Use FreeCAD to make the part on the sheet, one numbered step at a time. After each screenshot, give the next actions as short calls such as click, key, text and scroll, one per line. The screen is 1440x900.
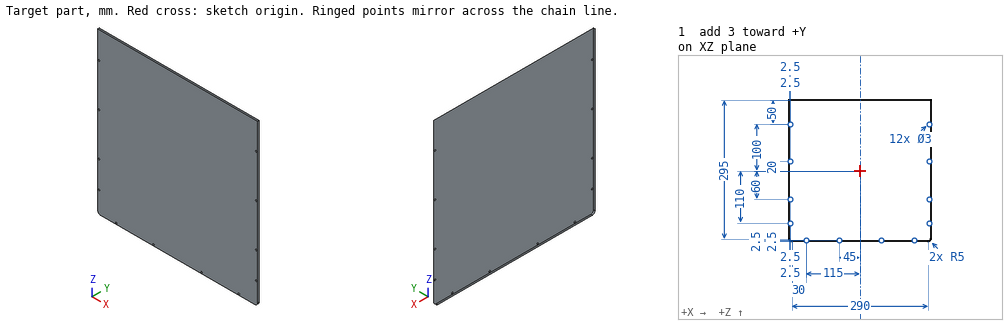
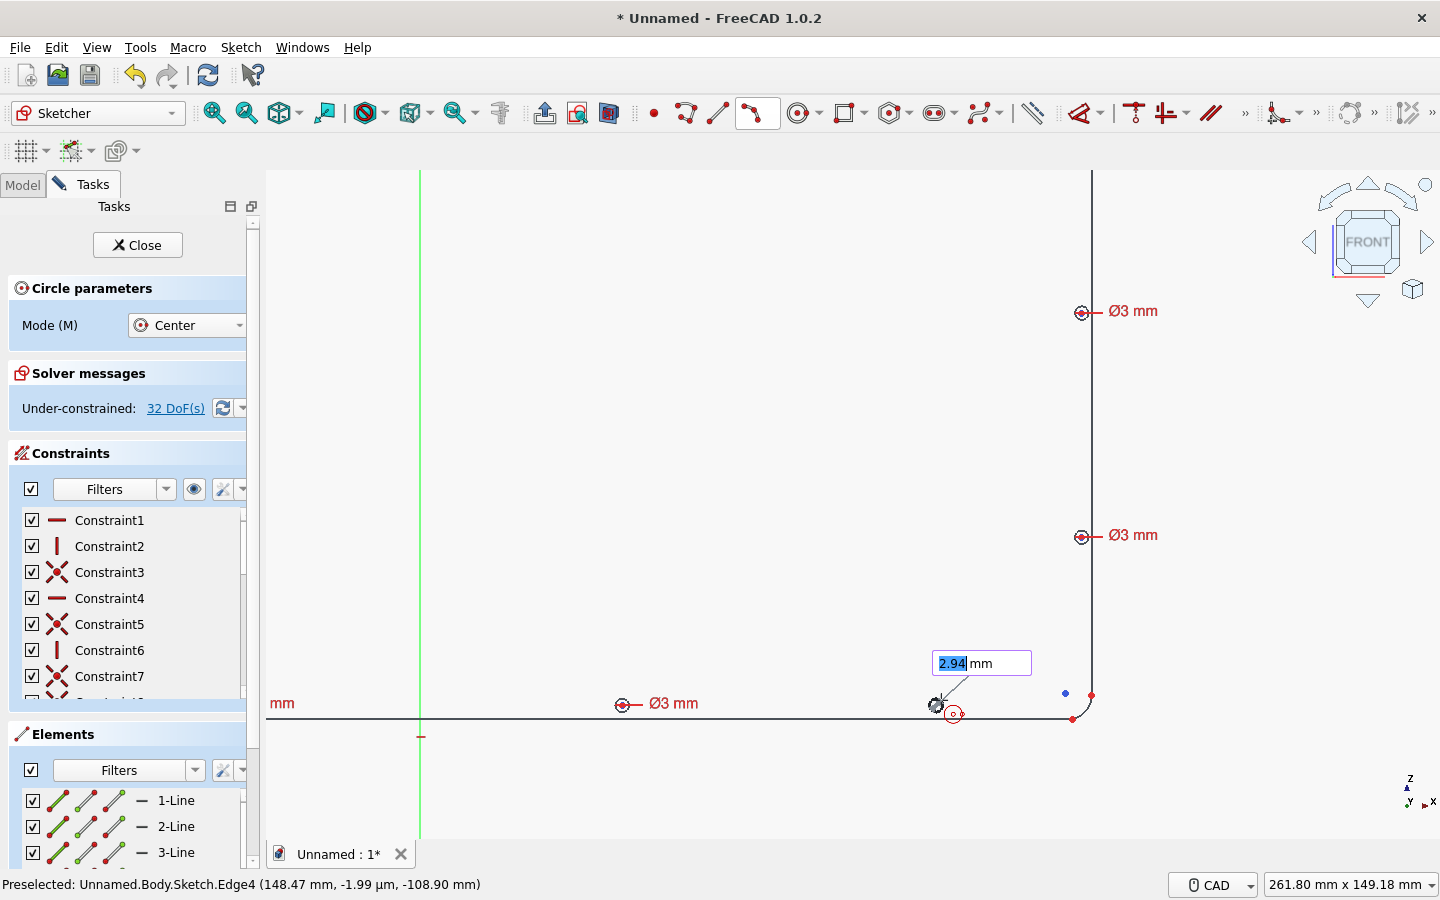
text(3)
key(Return)
key(Escape)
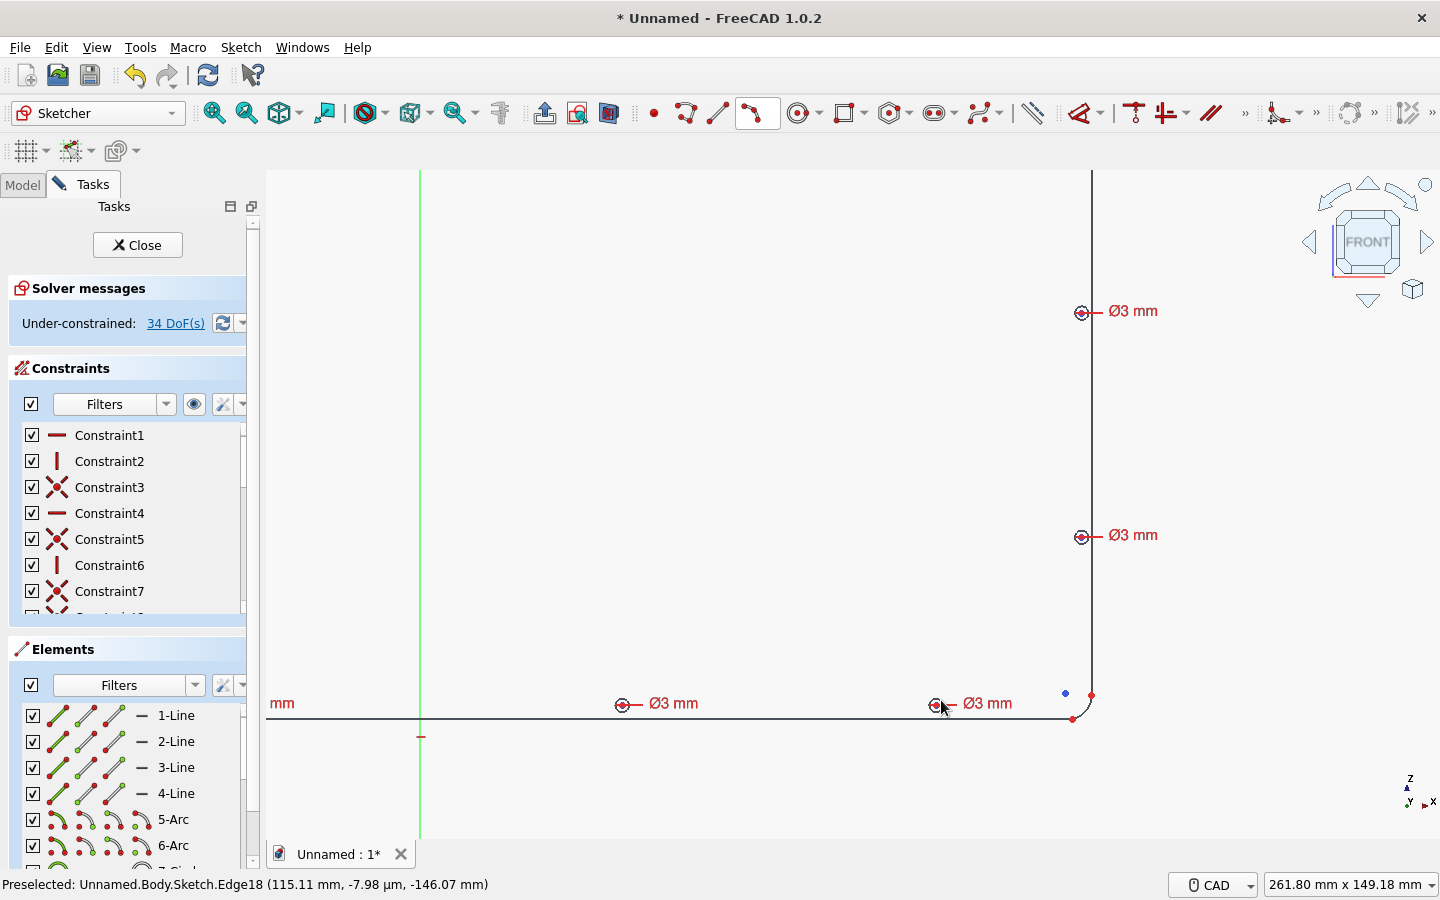
click(682, 719)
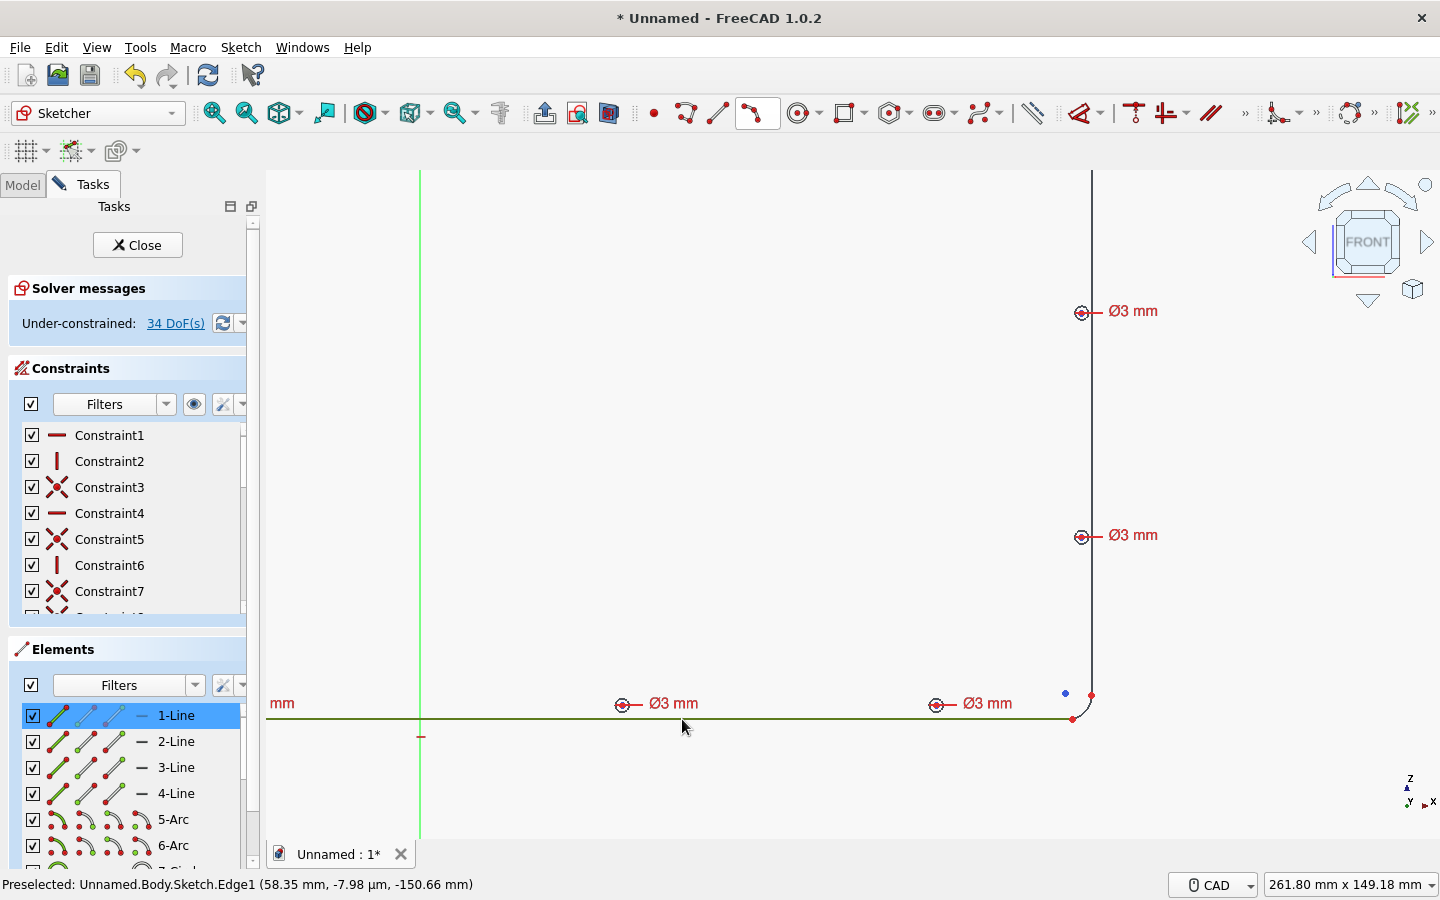
scroll(941, 703, down, 6)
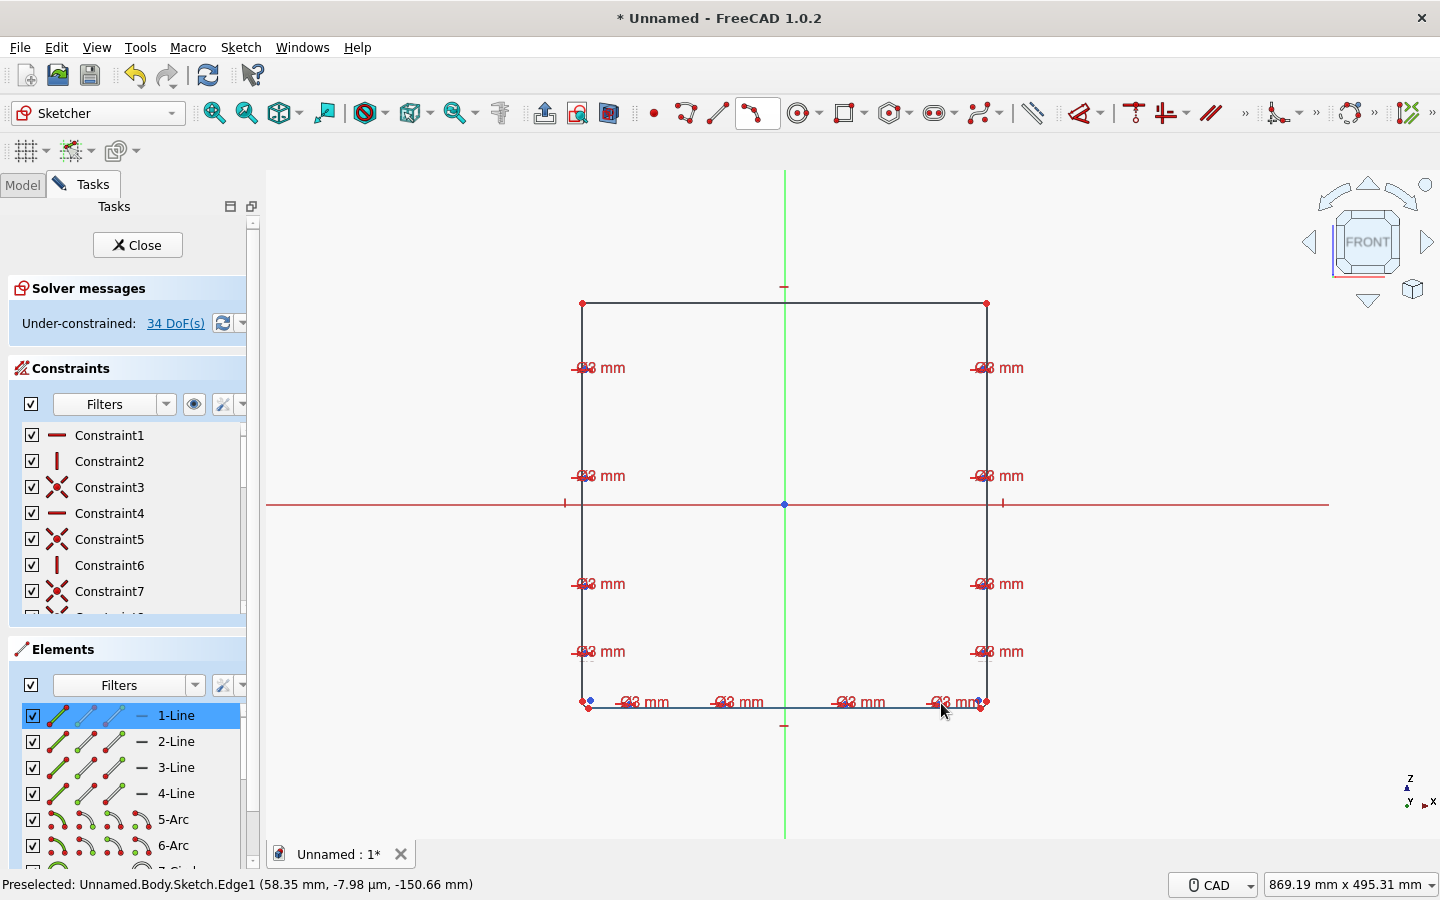
scroll(583, 704, up, 8)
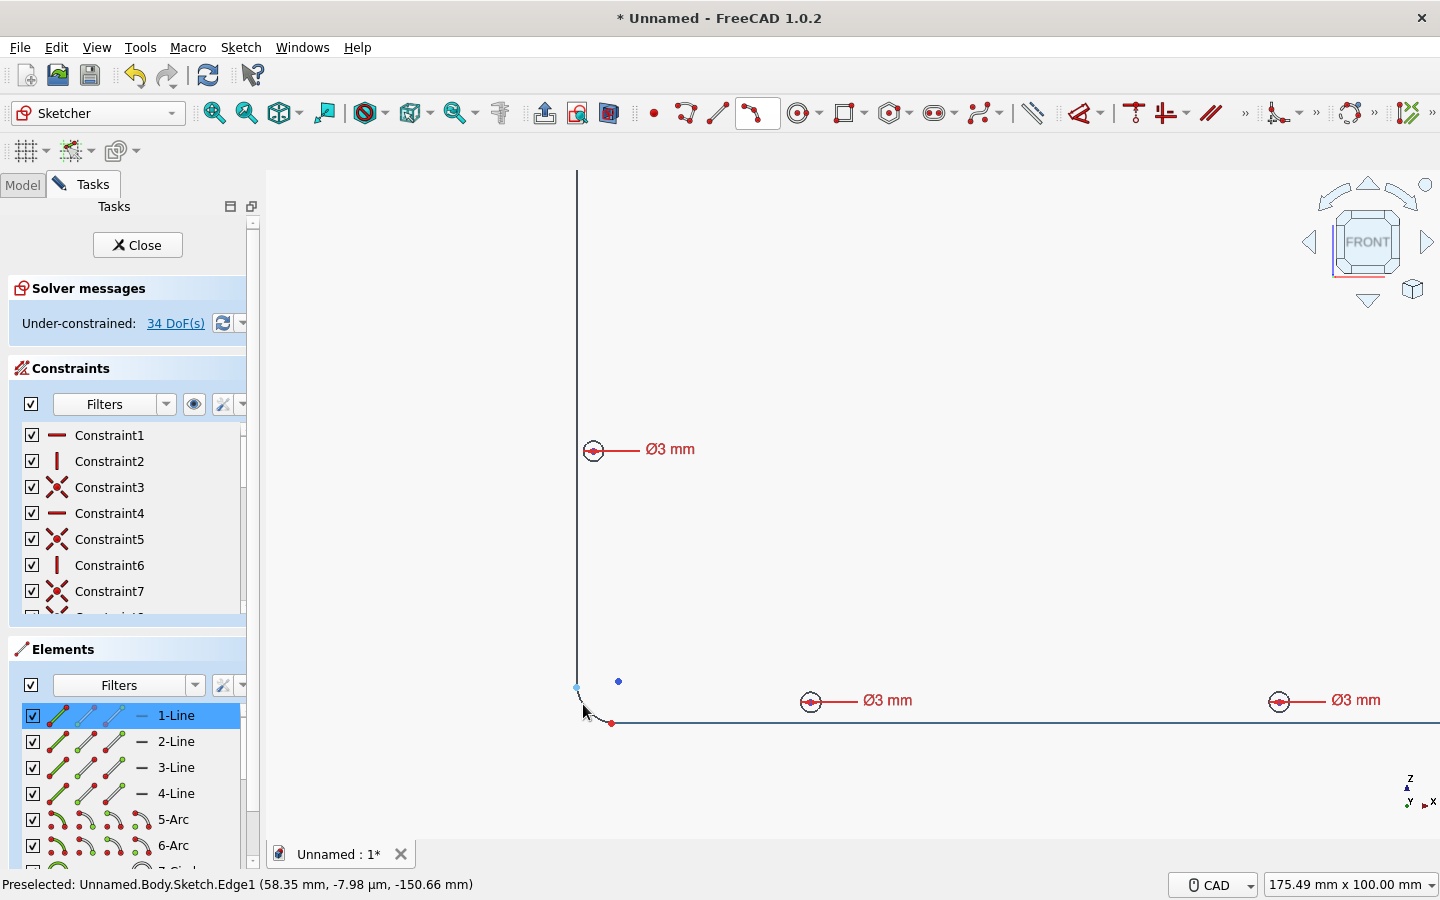
click(582, 703)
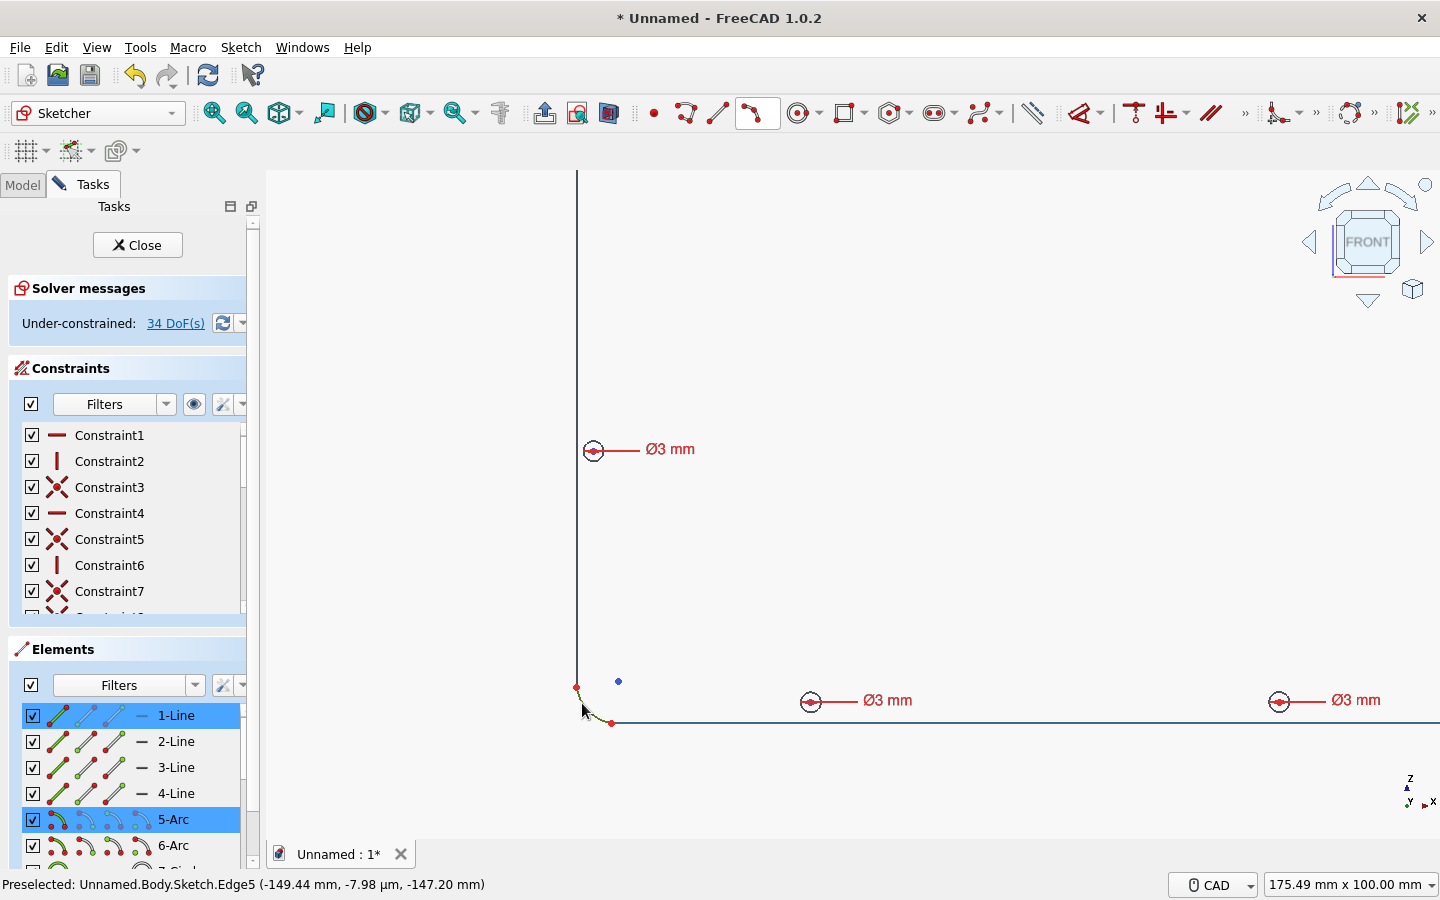
key(t)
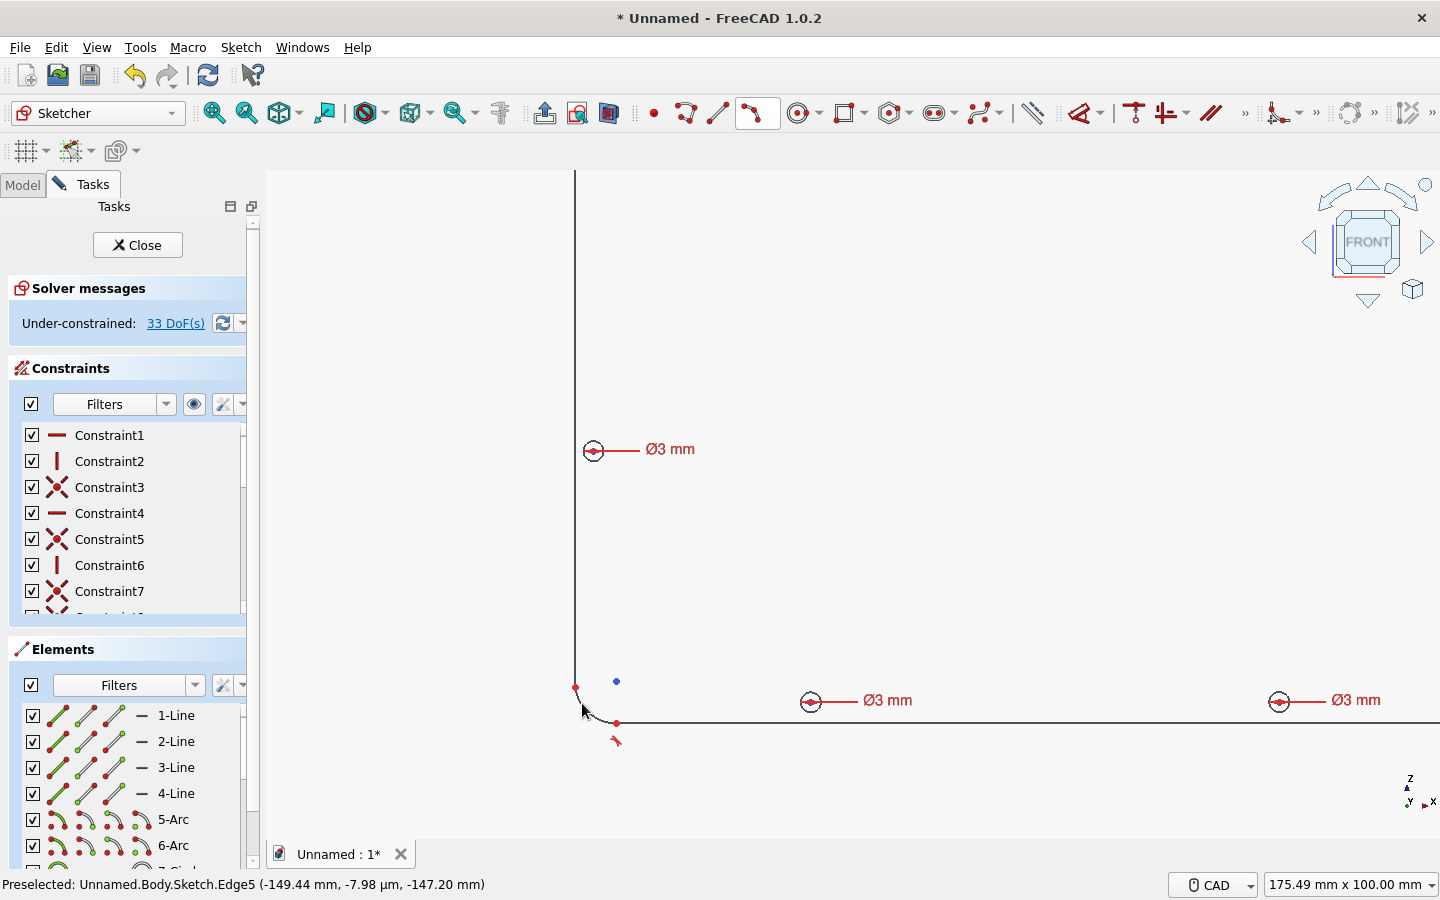
scroll(583, 704, down, 8)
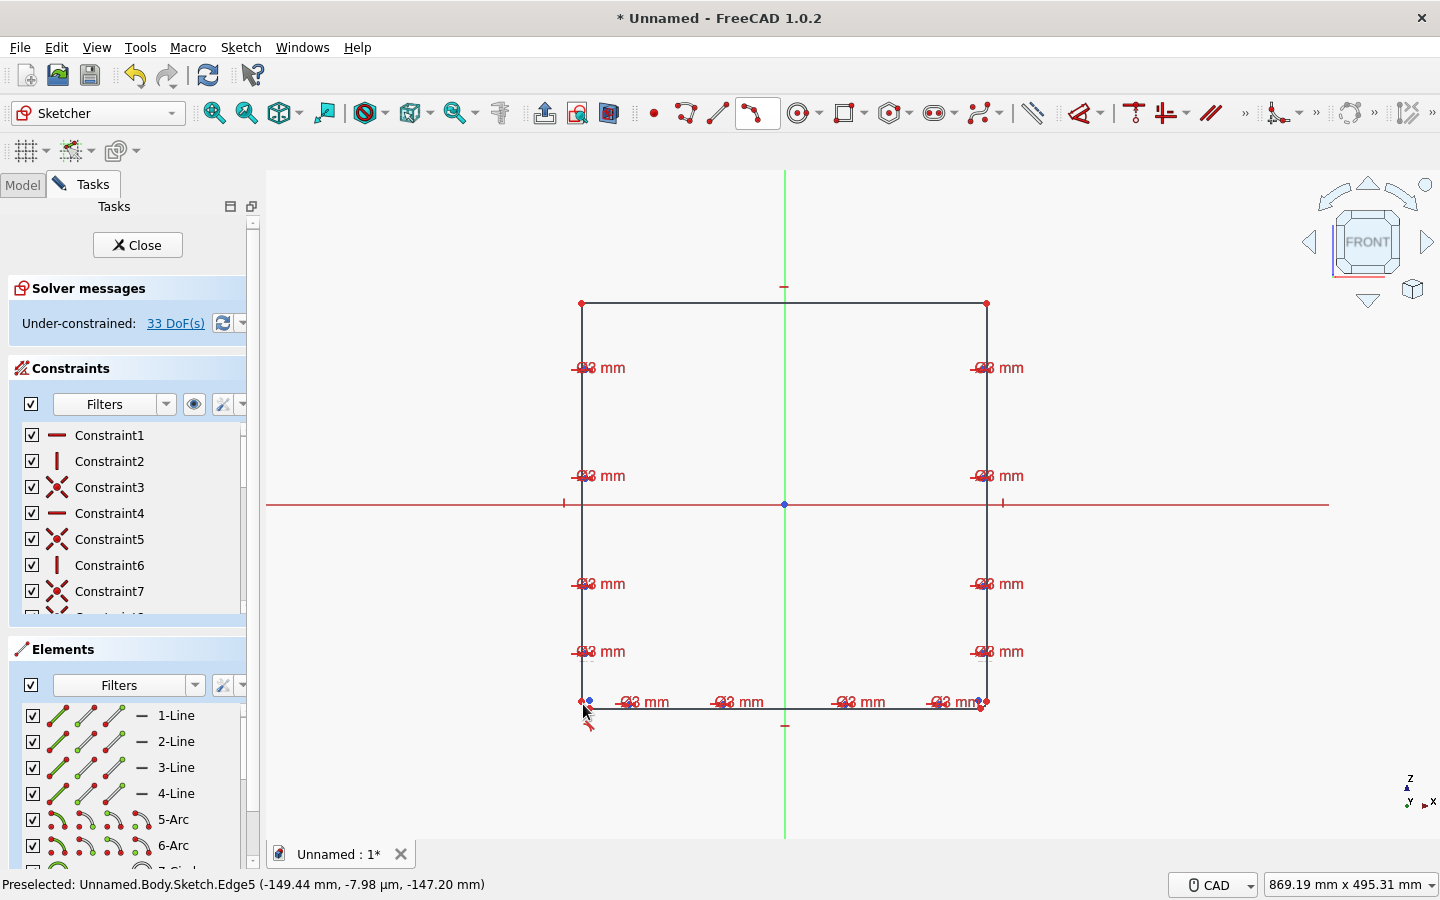
click(707, 709)